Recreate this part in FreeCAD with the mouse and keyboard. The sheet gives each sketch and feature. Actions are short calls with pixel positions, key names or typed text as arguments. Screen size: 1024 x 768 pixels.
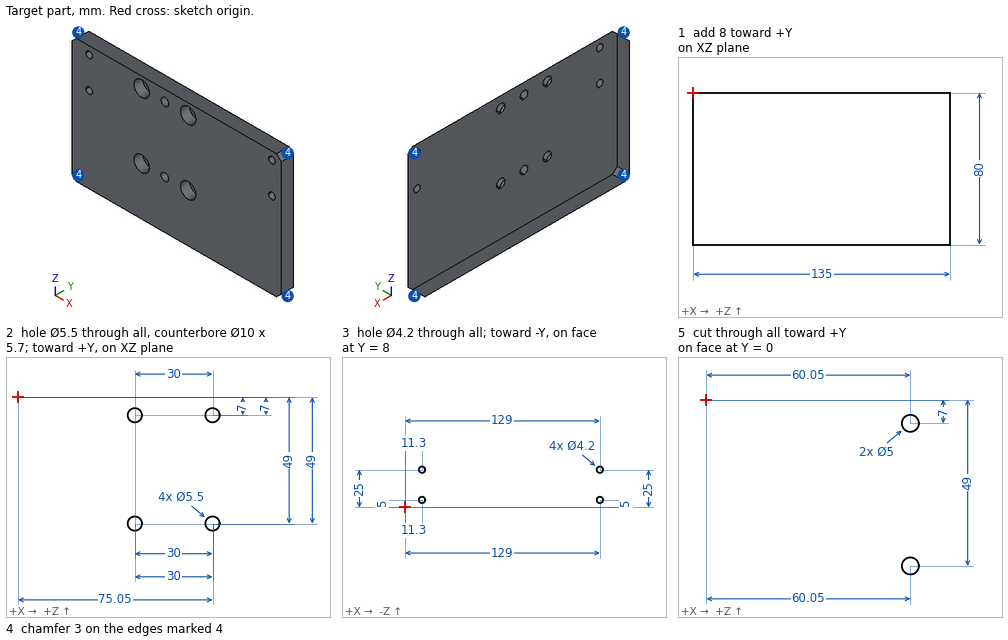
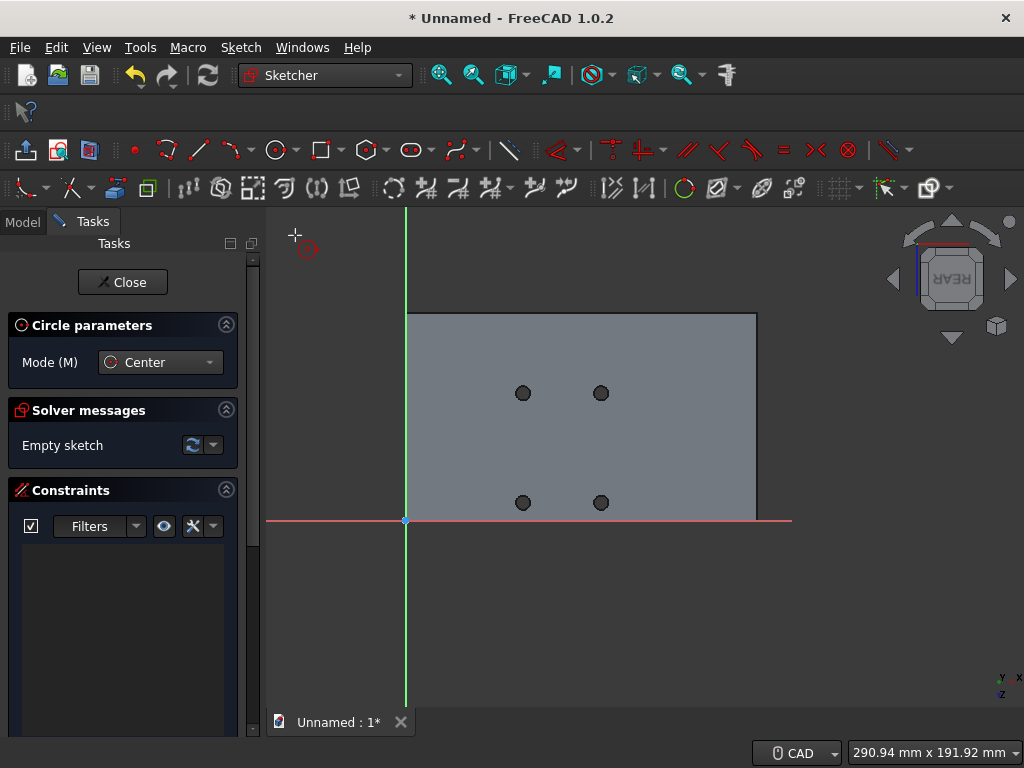
scroll(742, 456, up, 8)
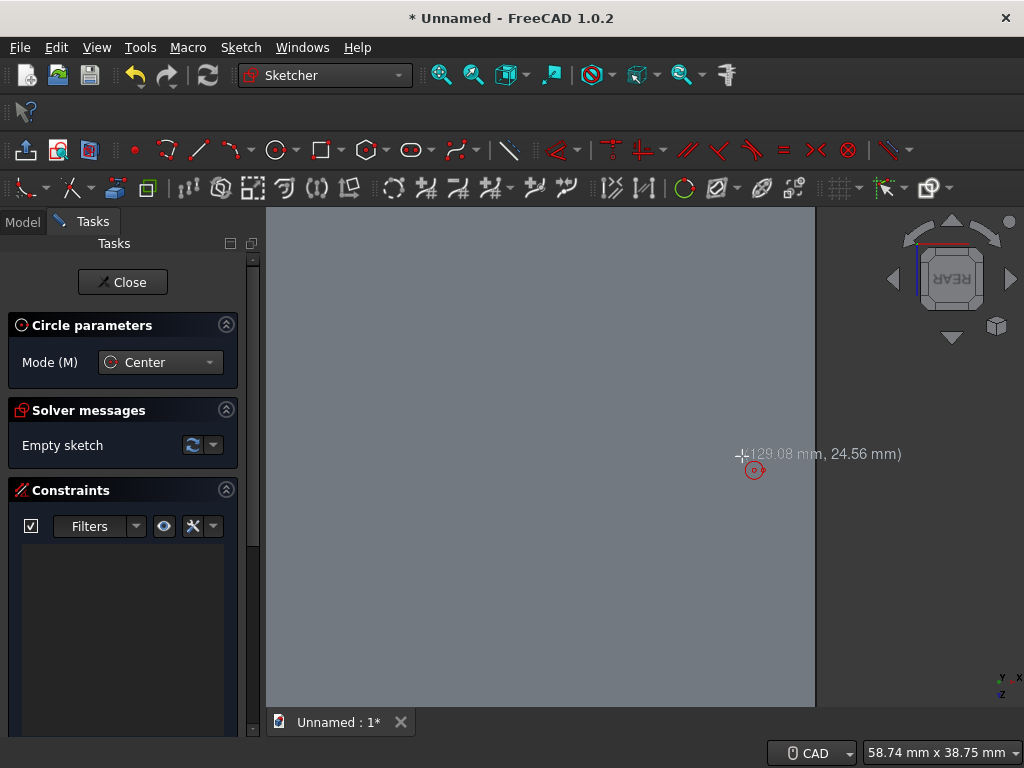
scroll(791, 410, down, 7)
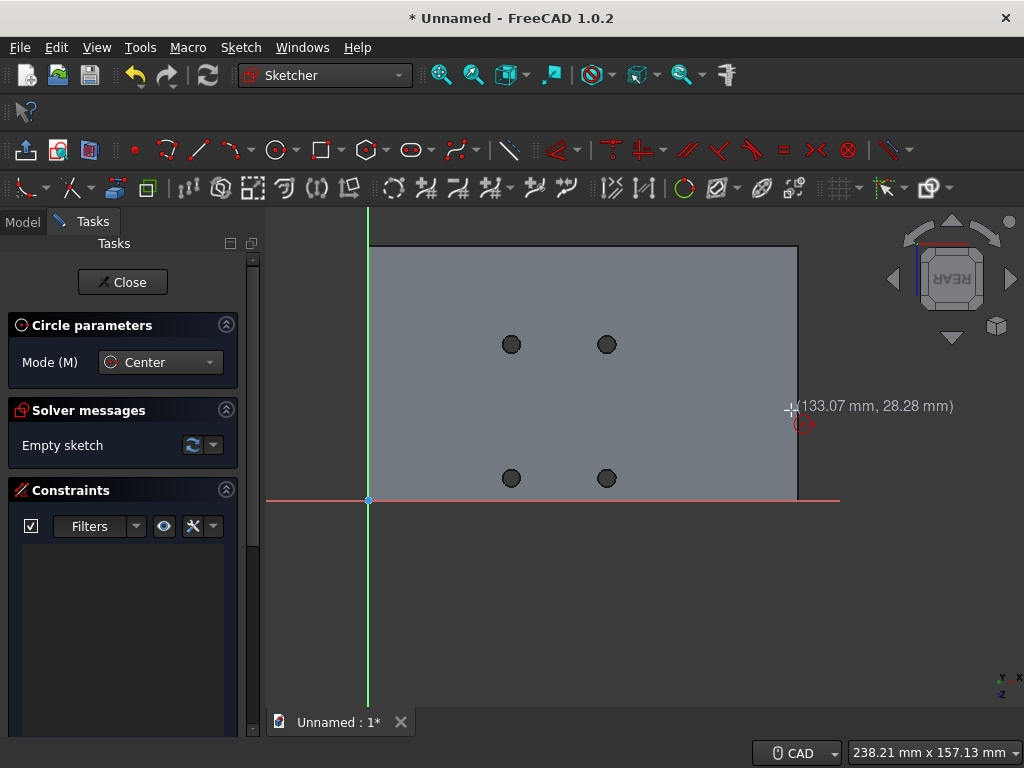
click(779, 421)
move(783, 416)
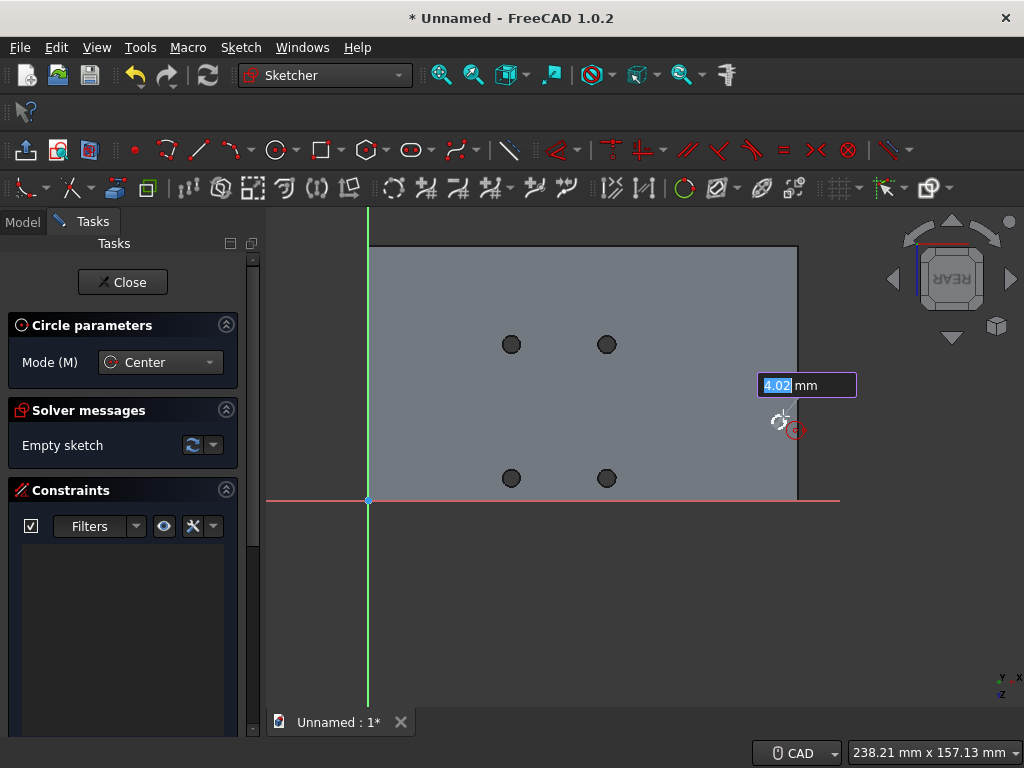
text(4.2)
key(Return)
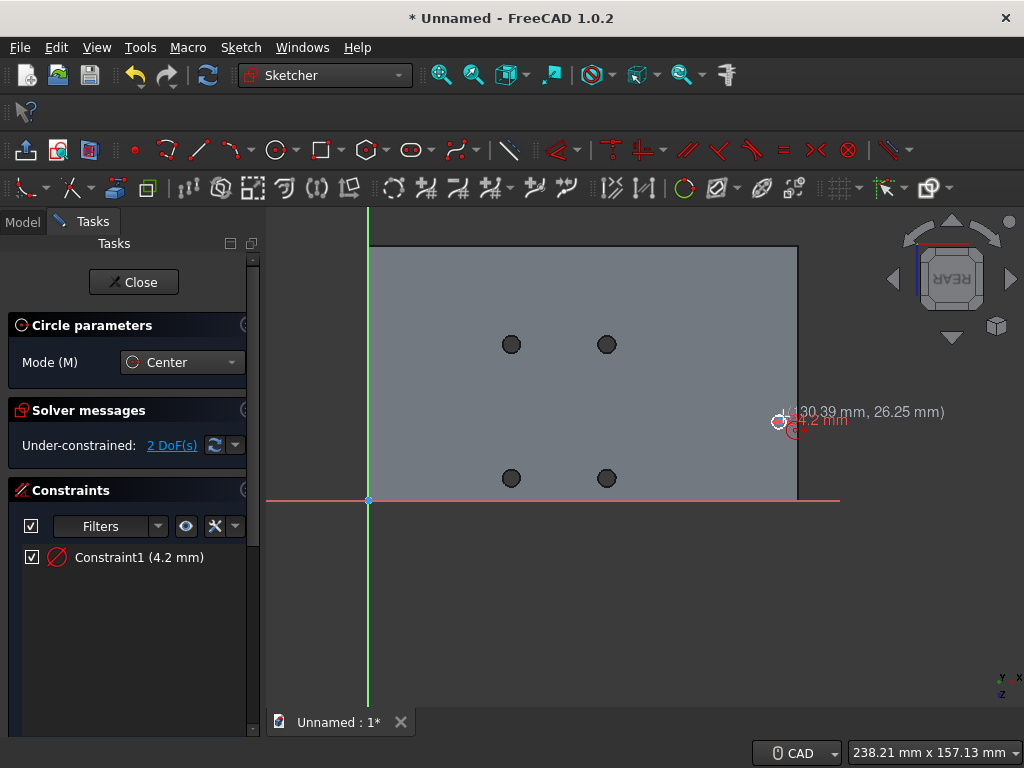
scroll(779, 485, up, 7)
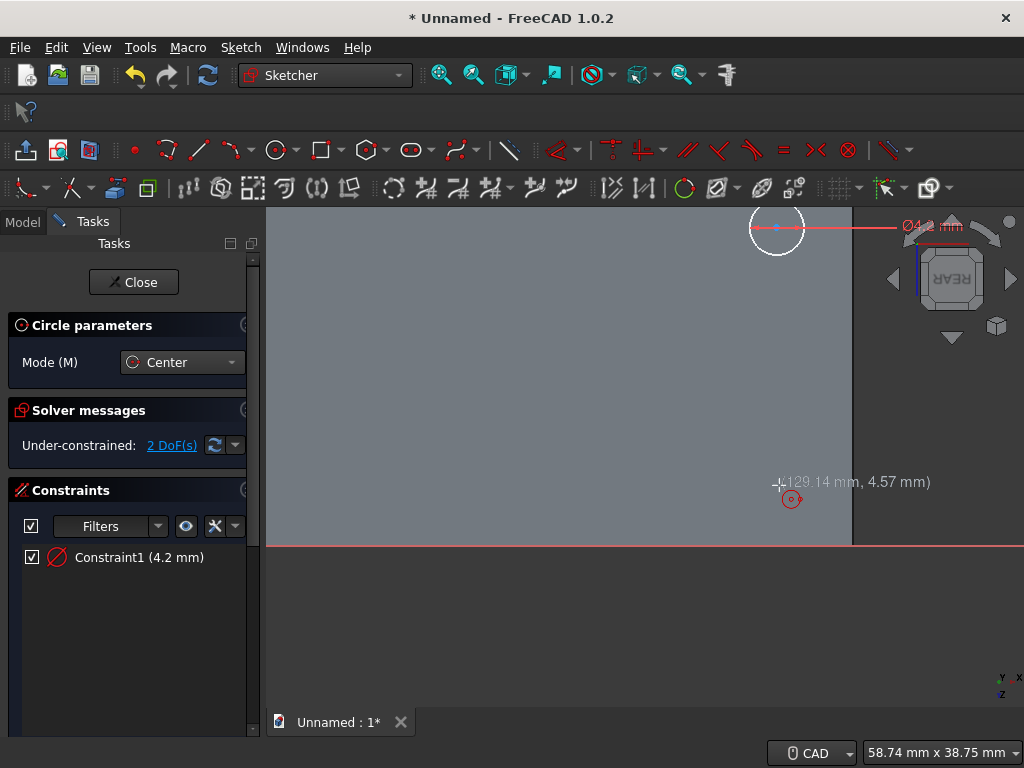
scroll(779, 485, down, 7)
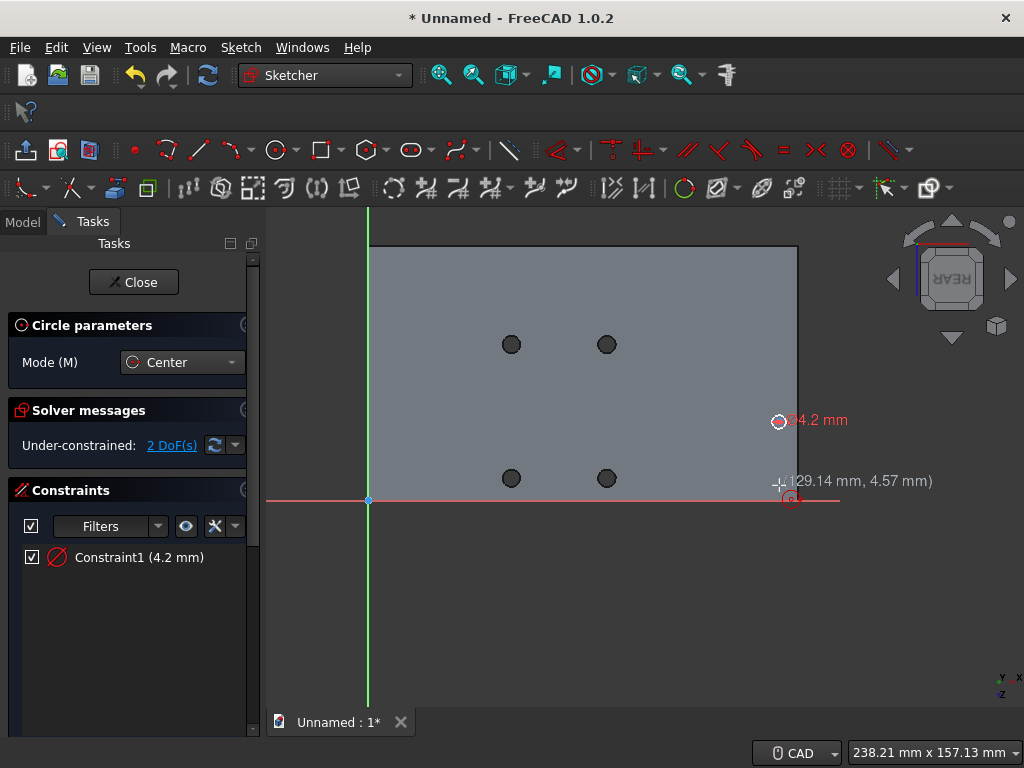
click(779, 485)
move(783, 480)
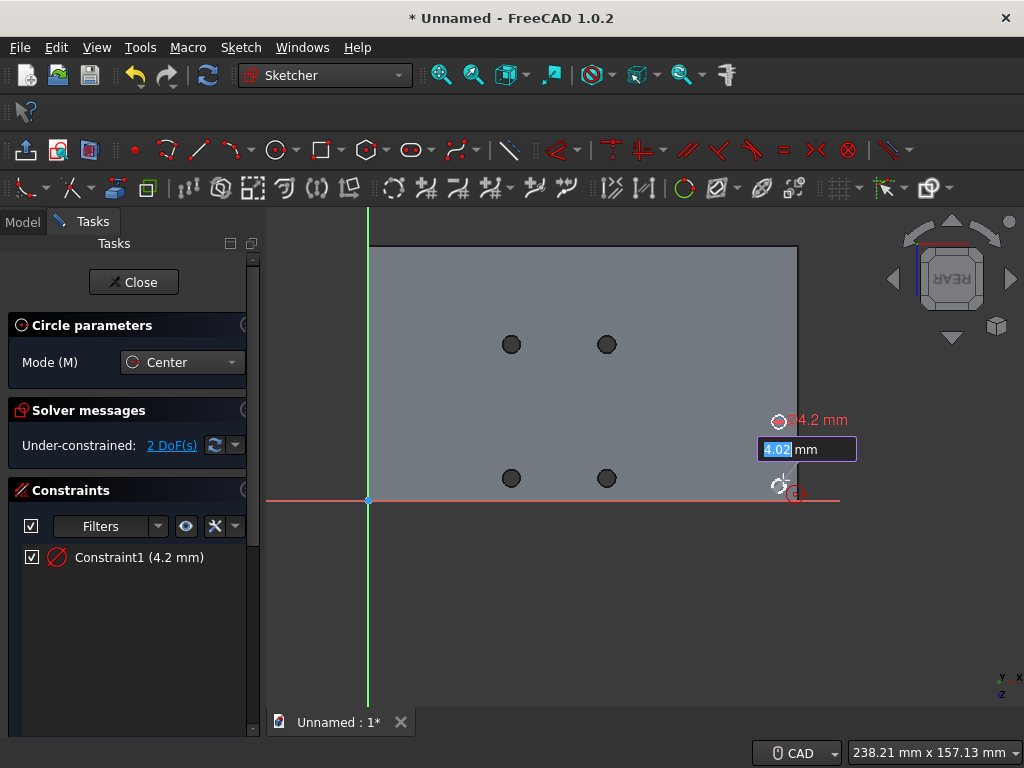
text(4.2)
key(Return)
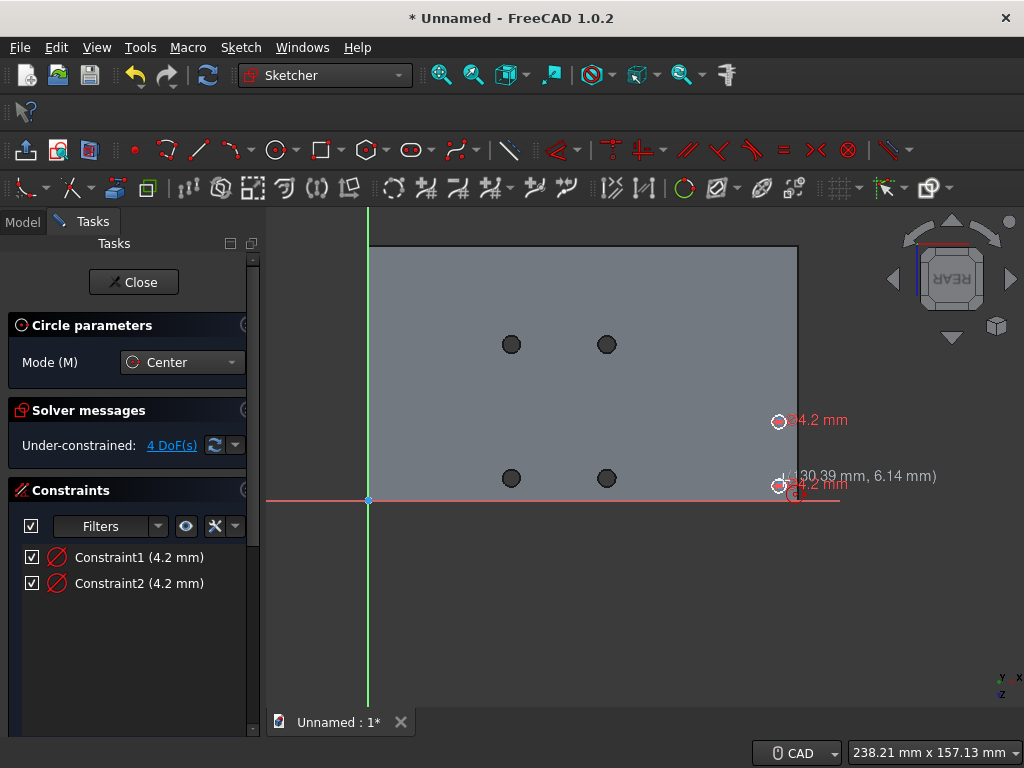
scroll(404, 421, up, 7)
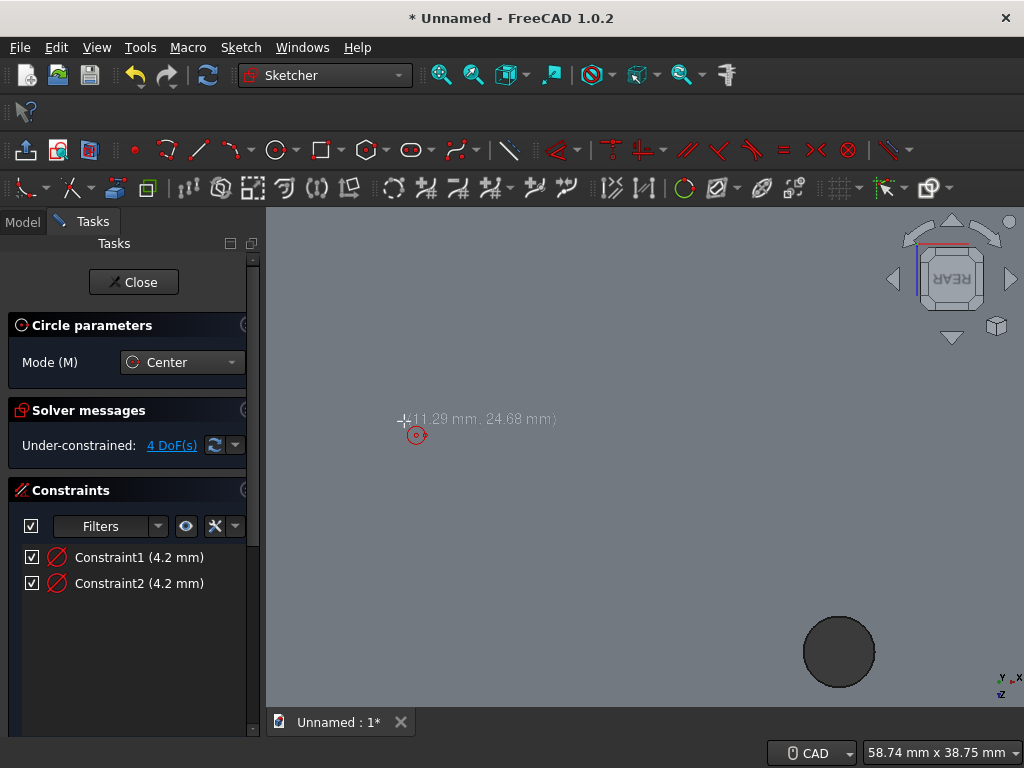
scroll(404, 421, down, 7)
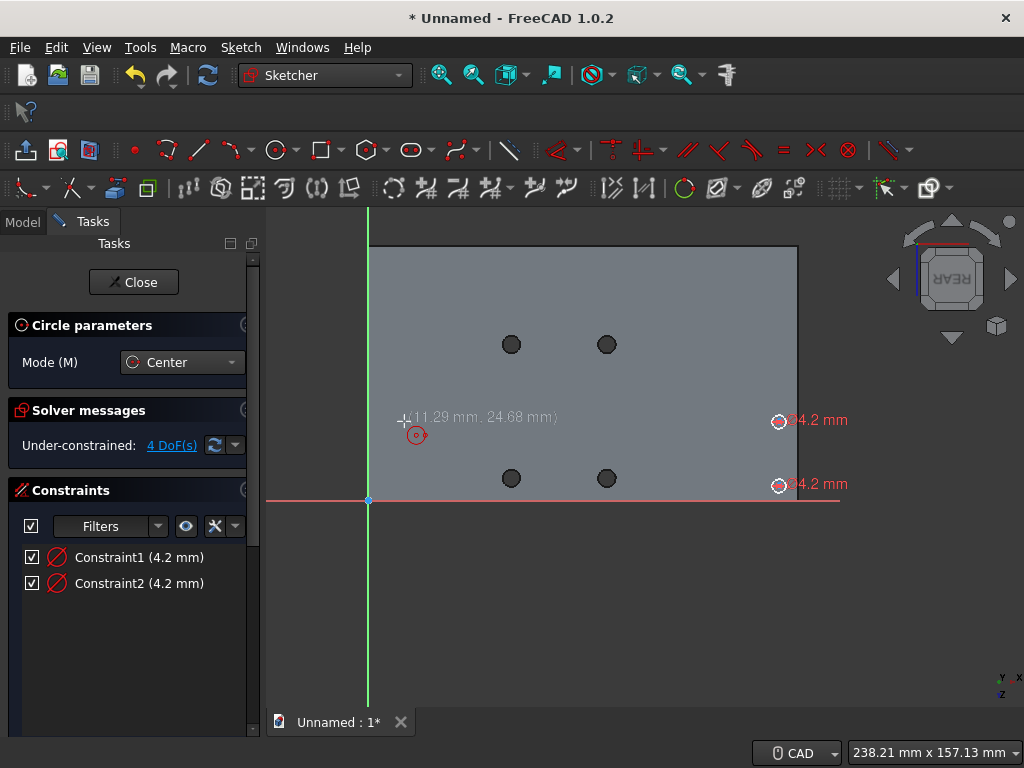
click(404, 421)
move(409, 416)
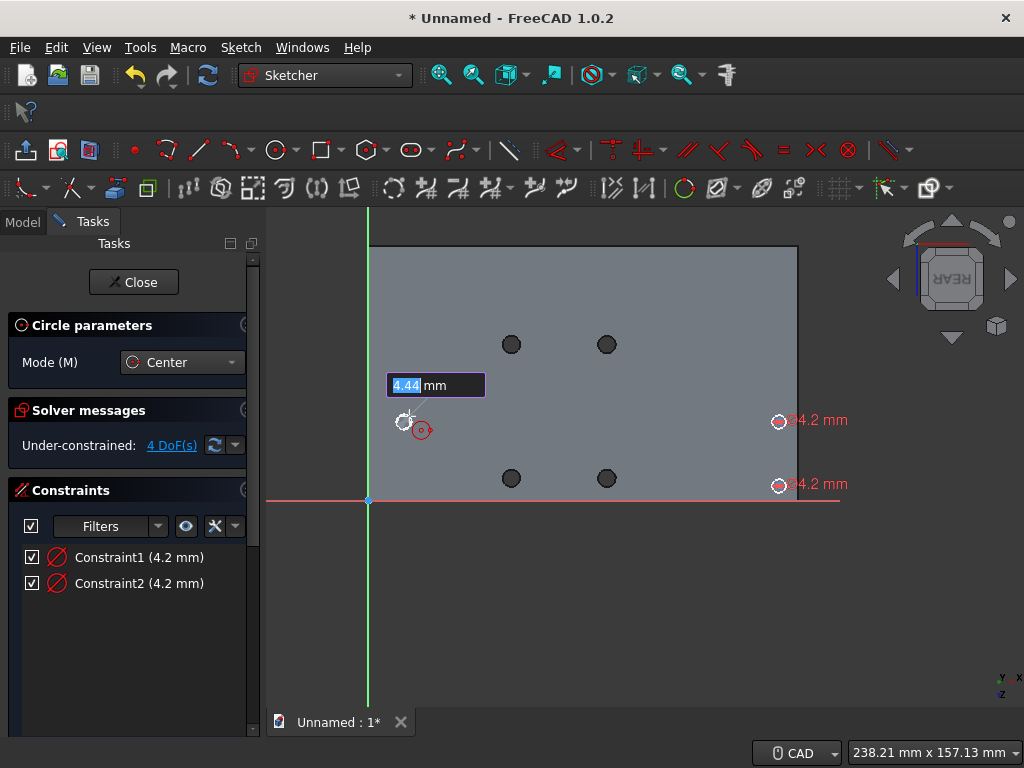
text(4.2)
key(Return)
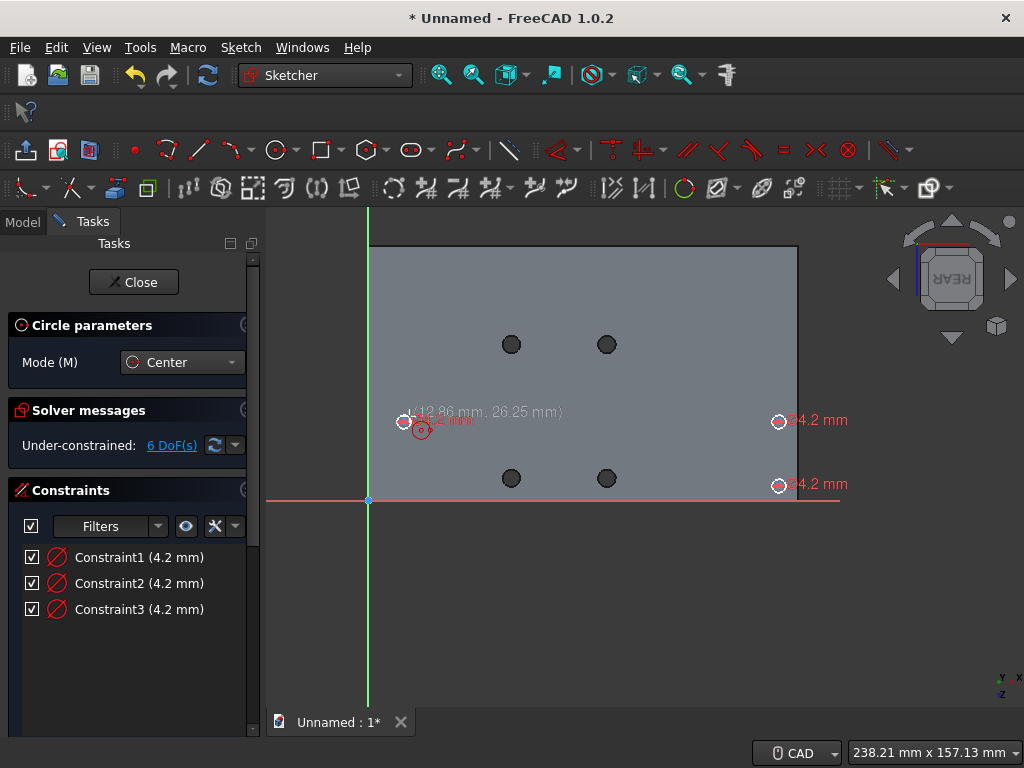
scroll(404, 485, up, 7)